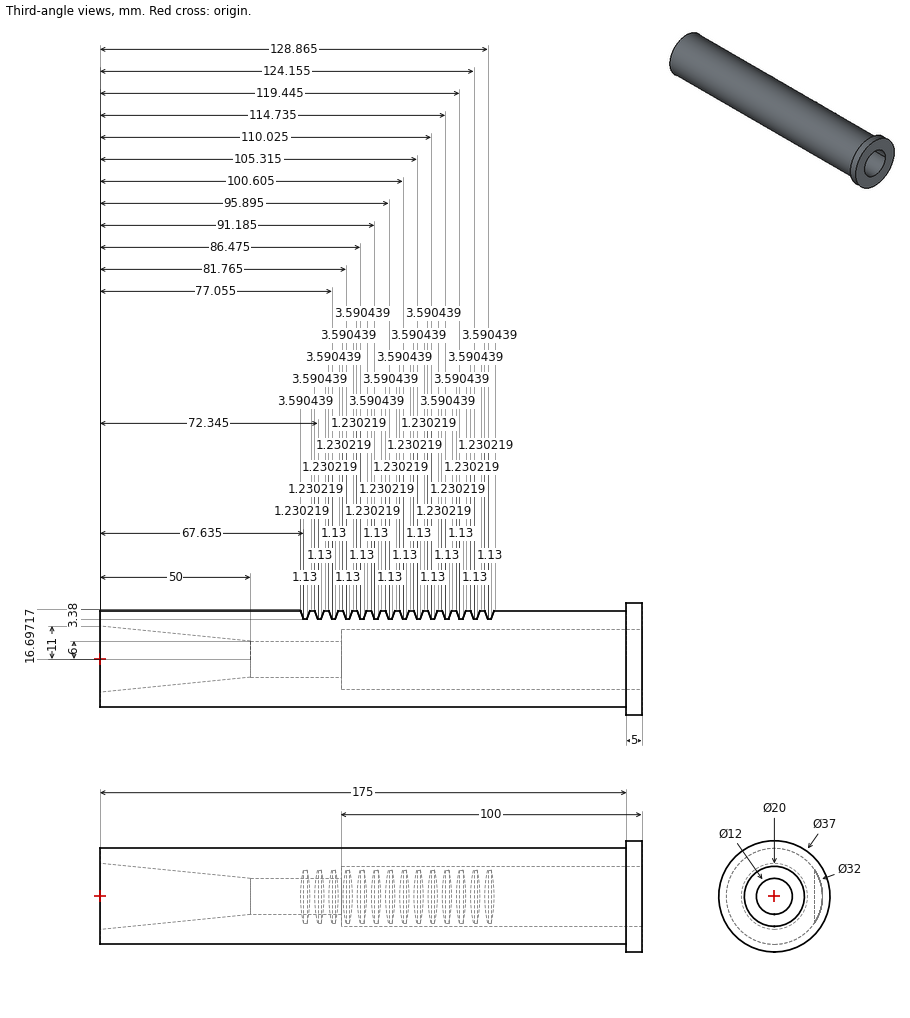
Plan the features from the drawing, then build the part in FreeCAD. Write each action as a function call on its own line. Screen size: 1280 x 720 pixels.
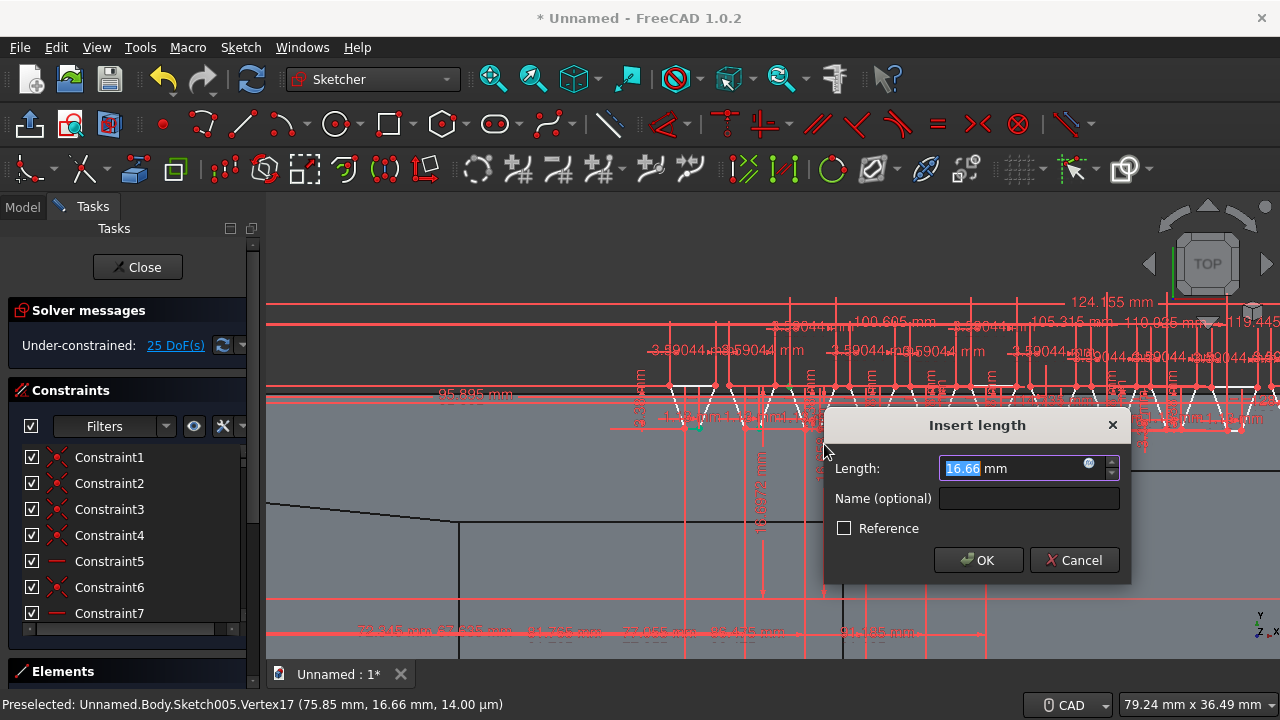
text(16.69717)
key(Return)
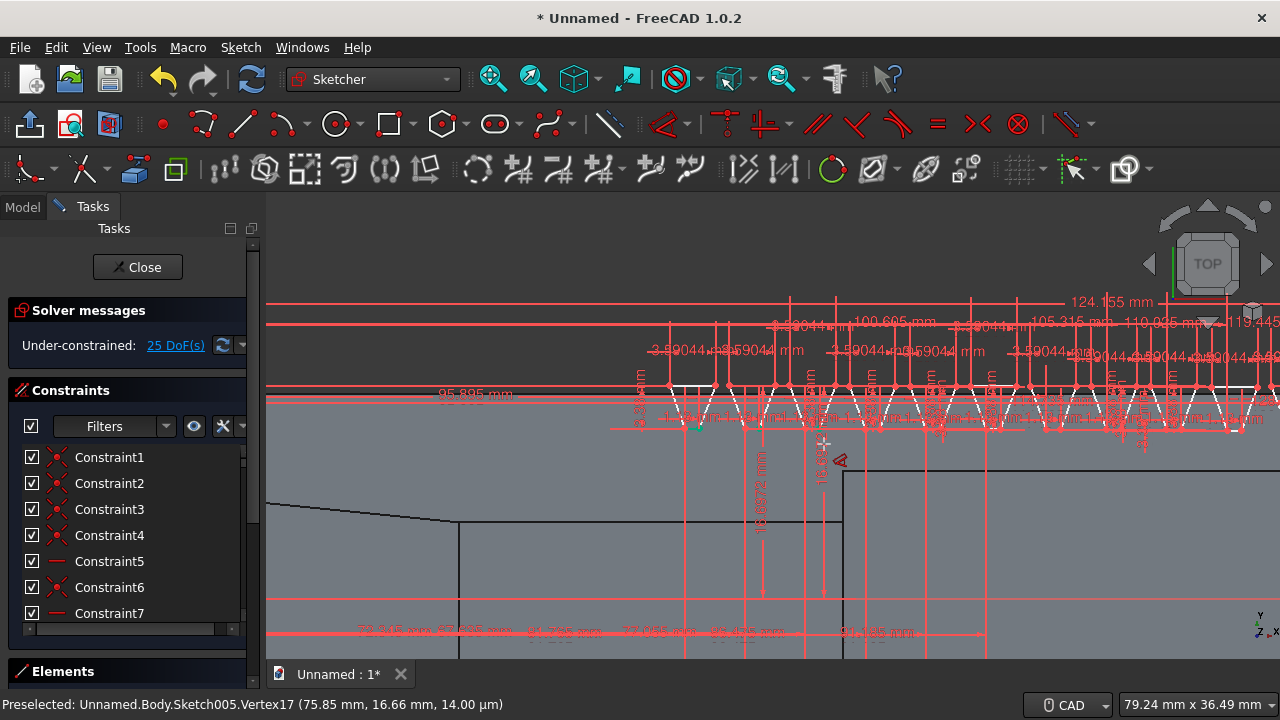
click(850, 386)
click(884, 493)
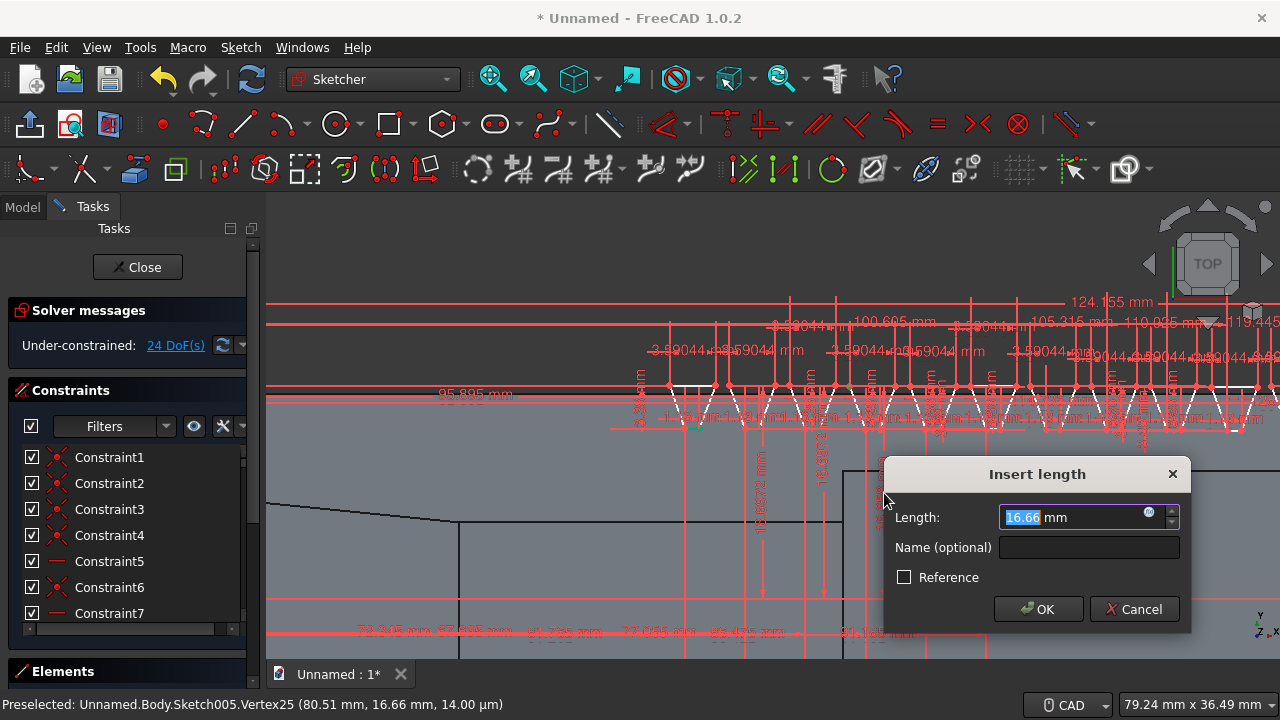
text(16.69717)
key(Return)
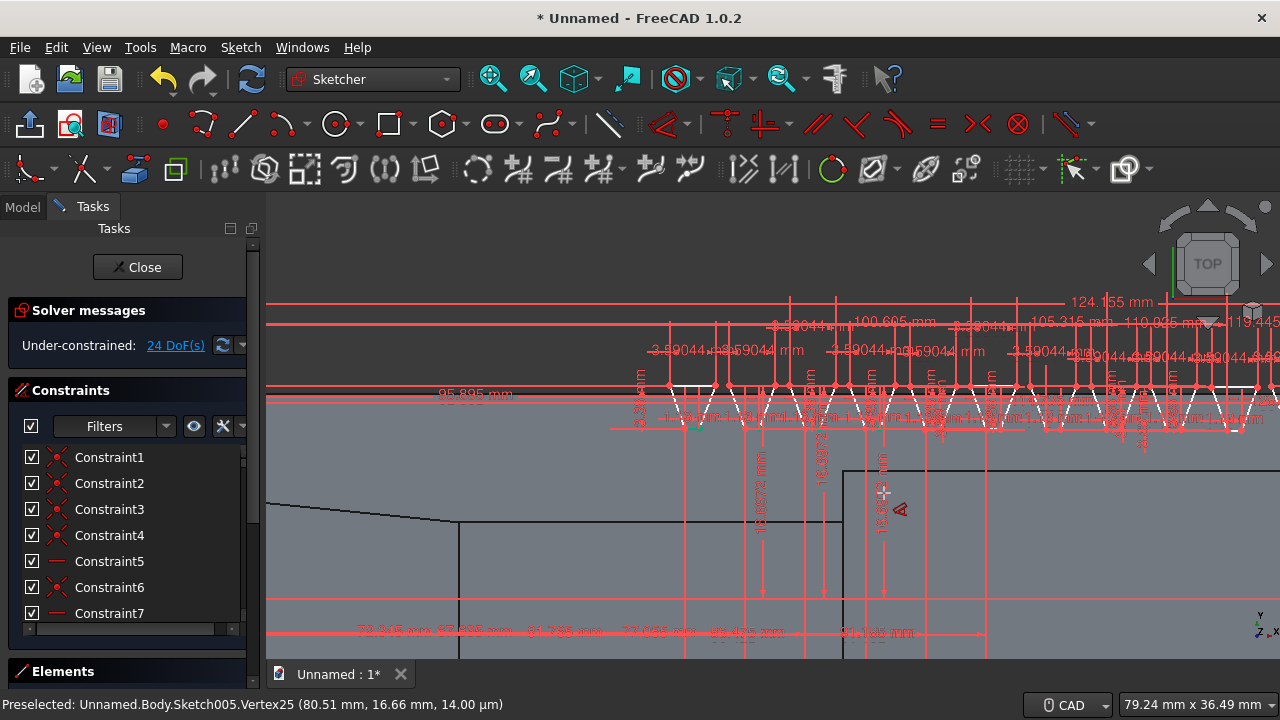
click(910, 387)
click(944, 444)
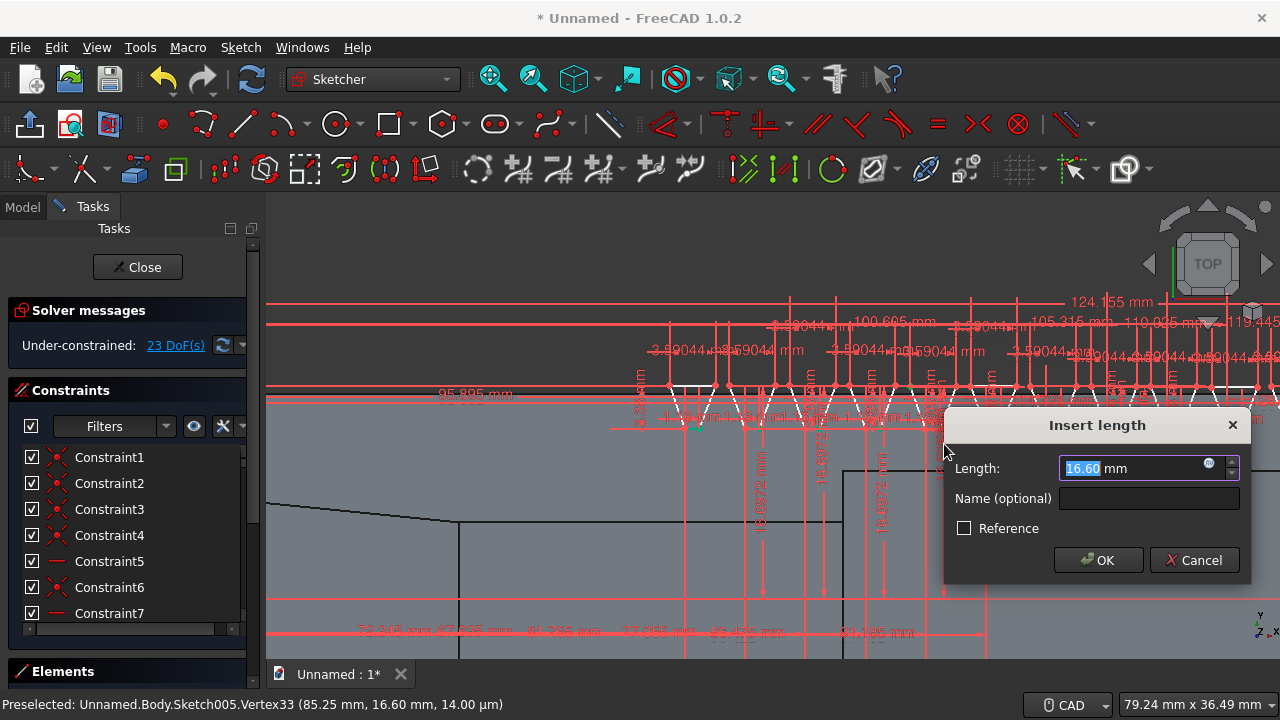
text(16.69717)
key(Return)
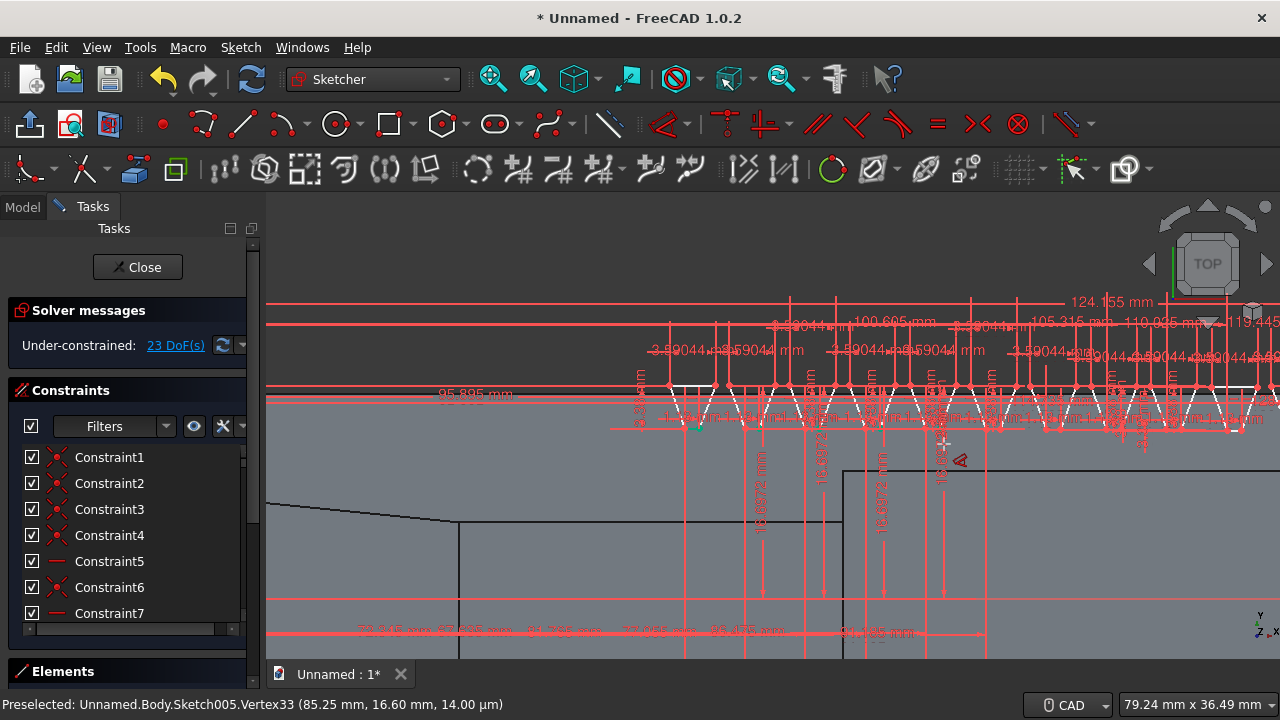
click(971, 386)
click(1005, 493)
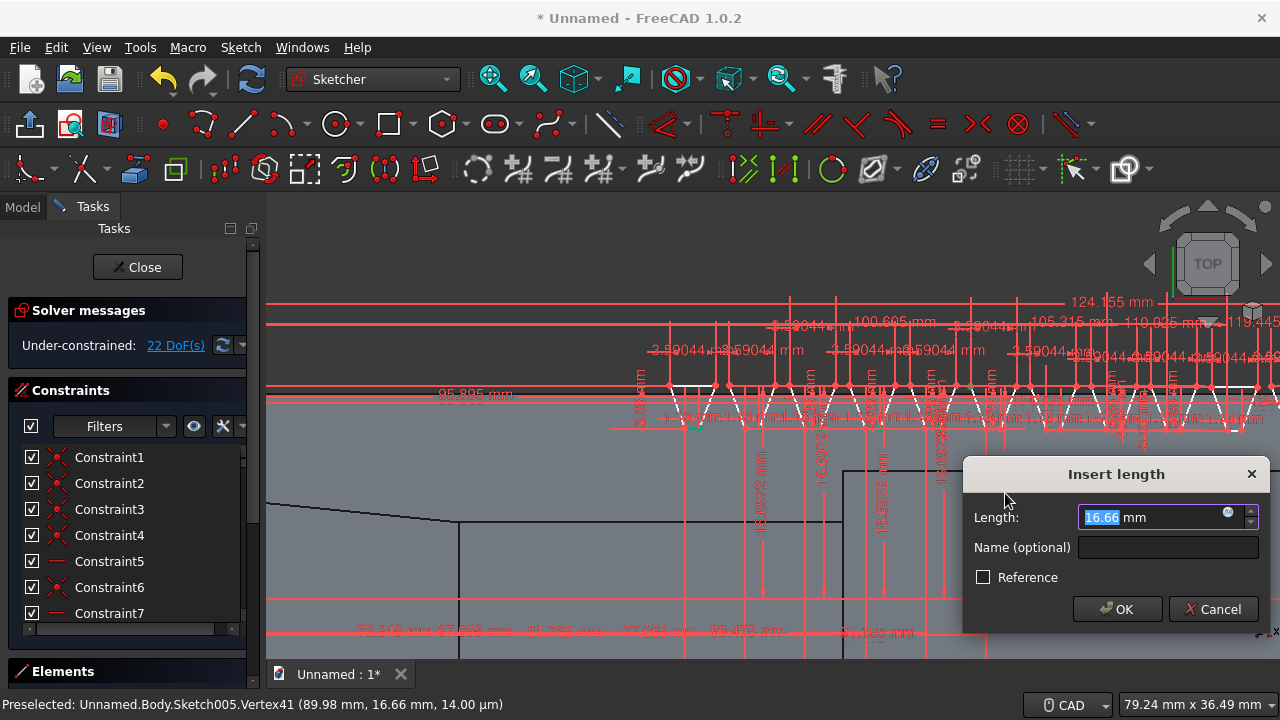
text(16.69717)
key(Return)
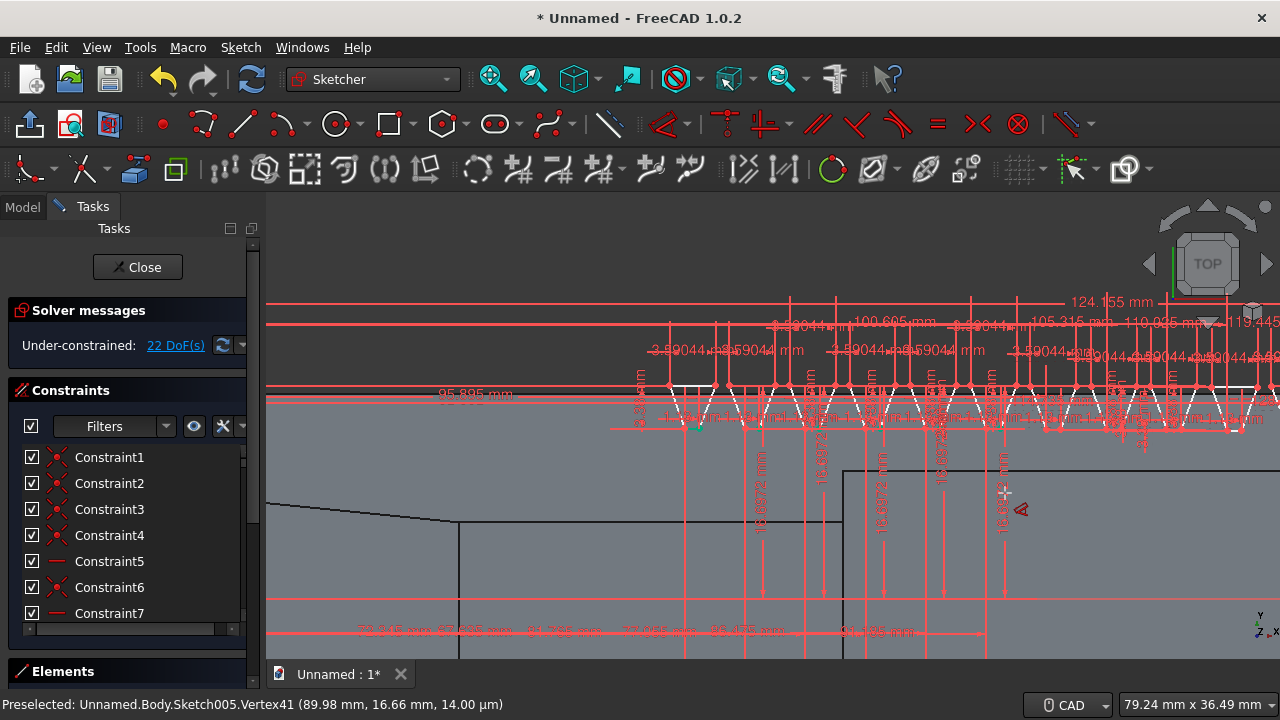
click(1030, 386)
click(1064, 444)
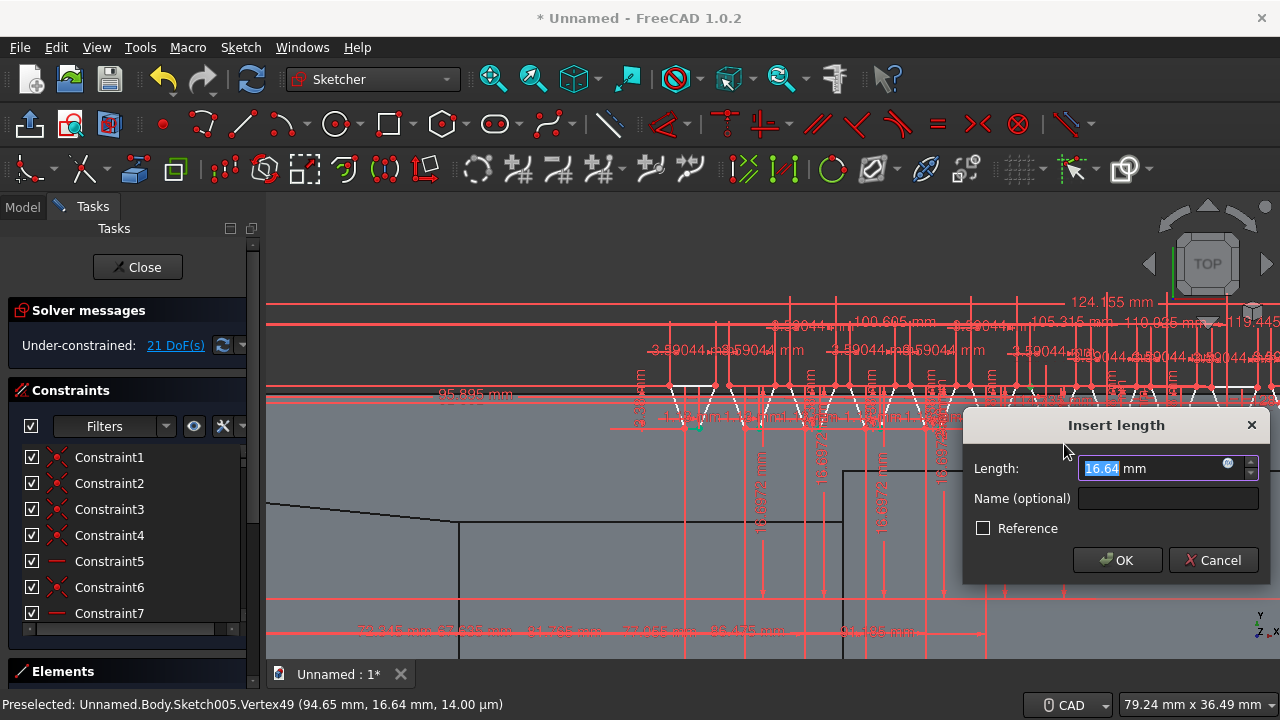
text(16.69717)
key(Return)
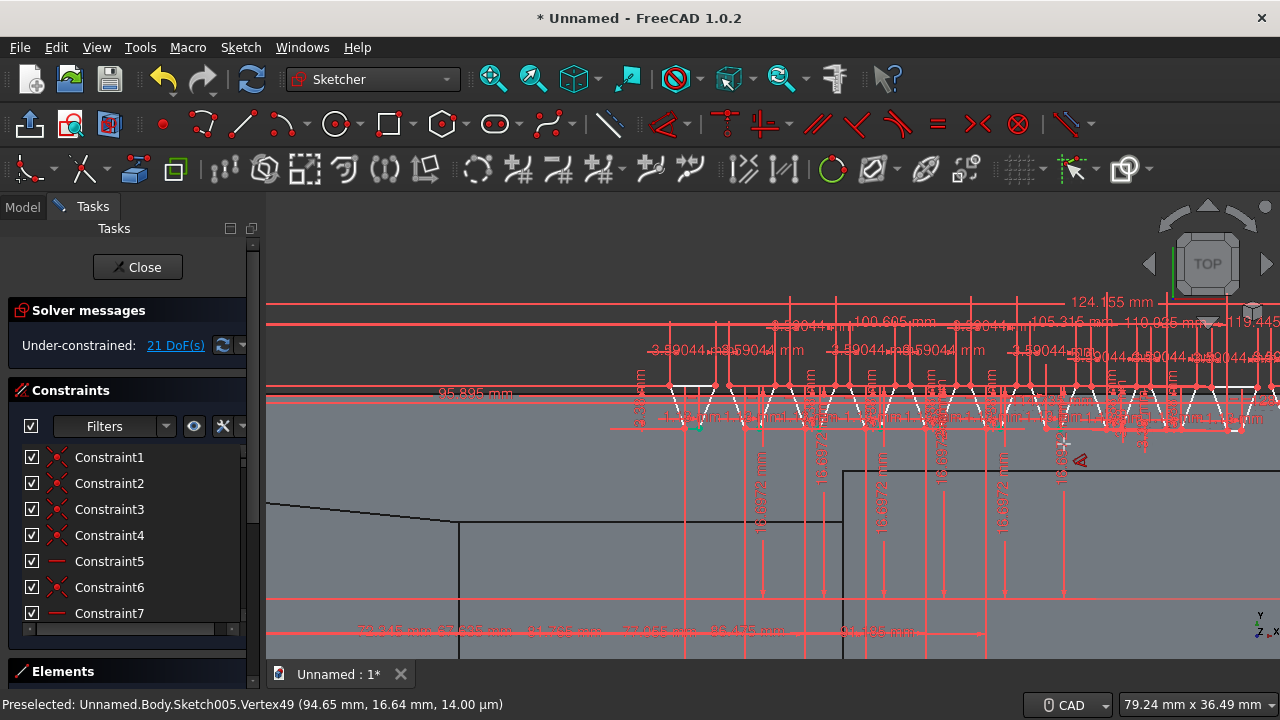
click(1091, 386)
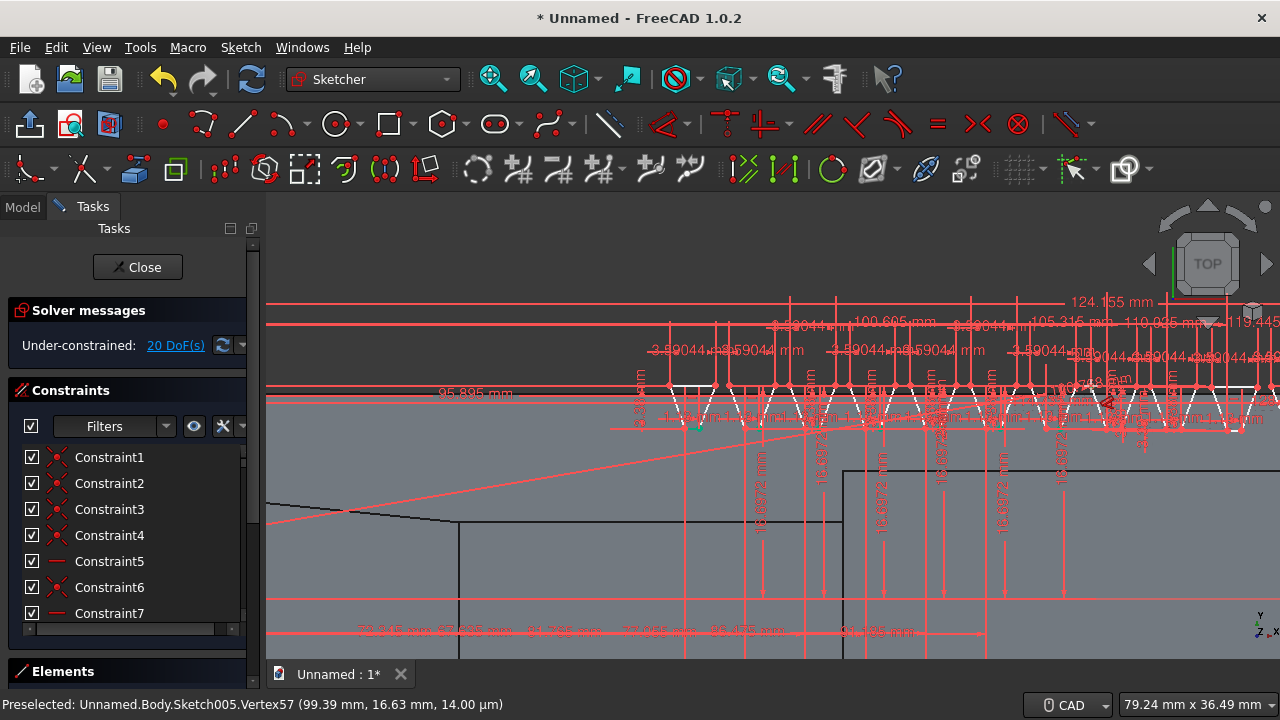
key(Escape)
key(Escape)